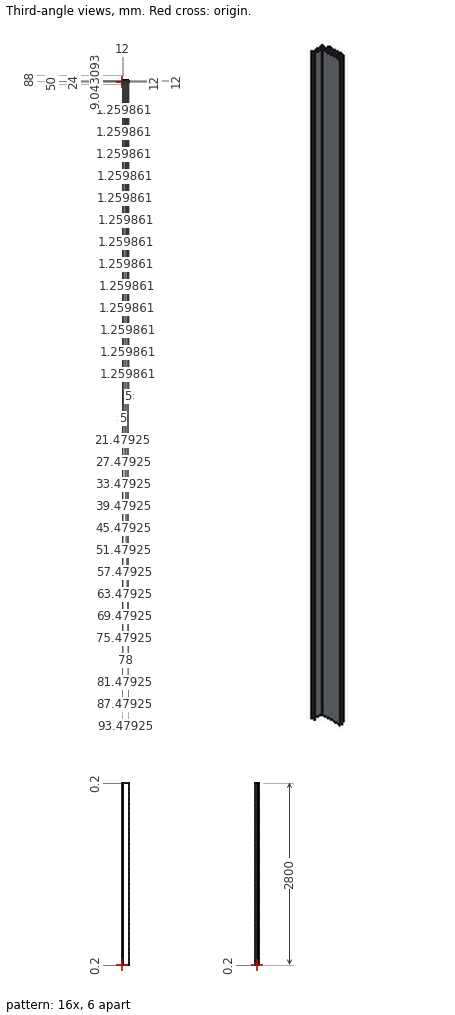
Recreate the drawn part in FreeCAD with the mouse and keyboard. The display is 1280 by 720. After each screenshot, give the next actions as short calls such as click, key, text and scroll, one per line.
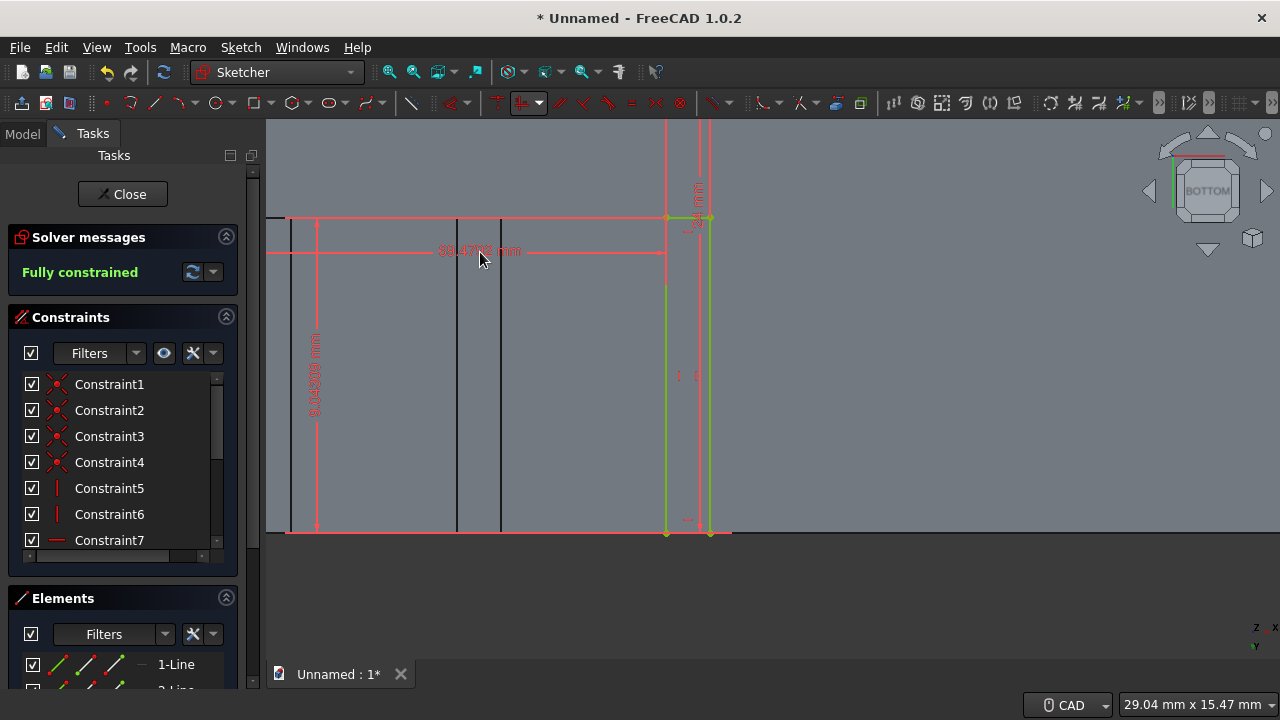
click(123, 194)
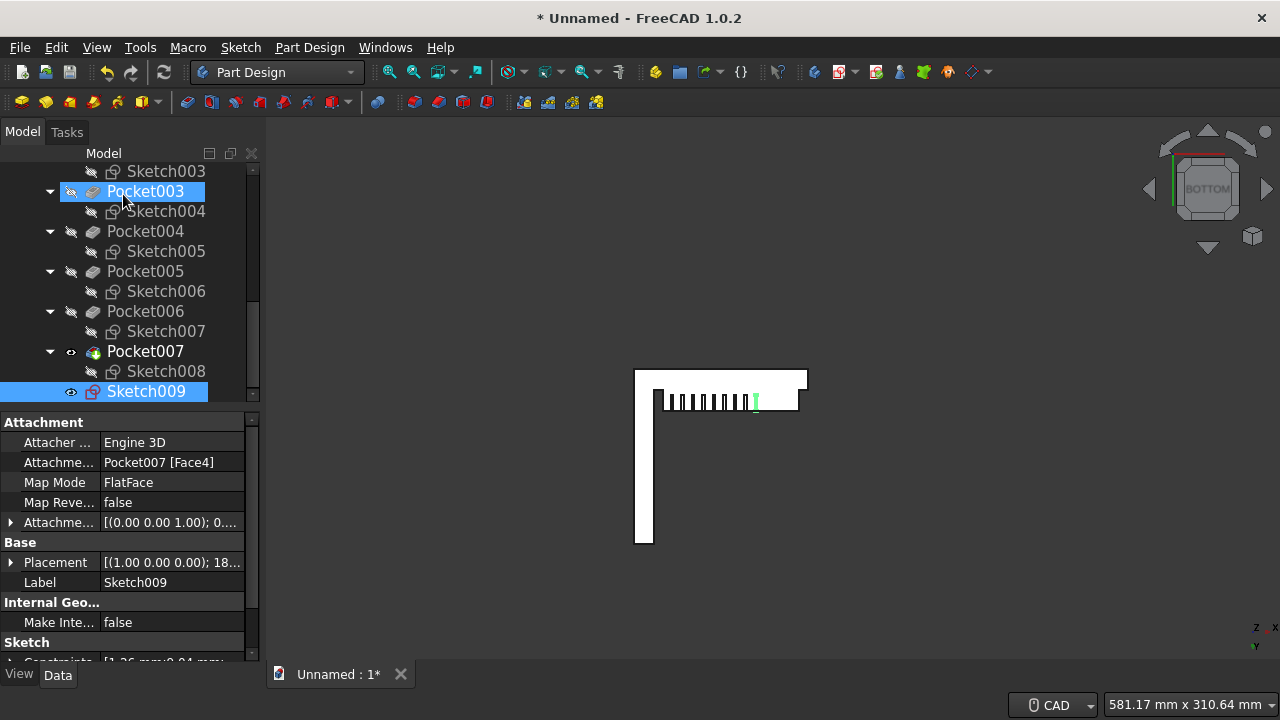
click(188, 102)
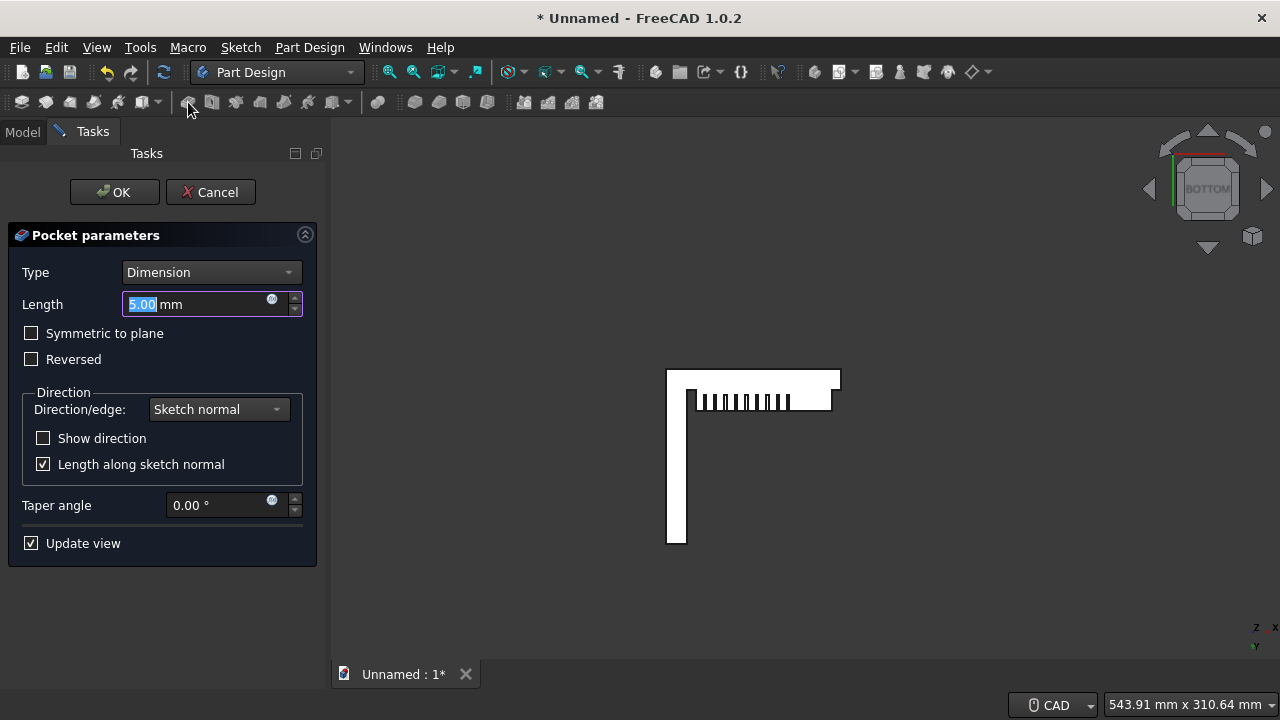
text(0.2)
key(Tab)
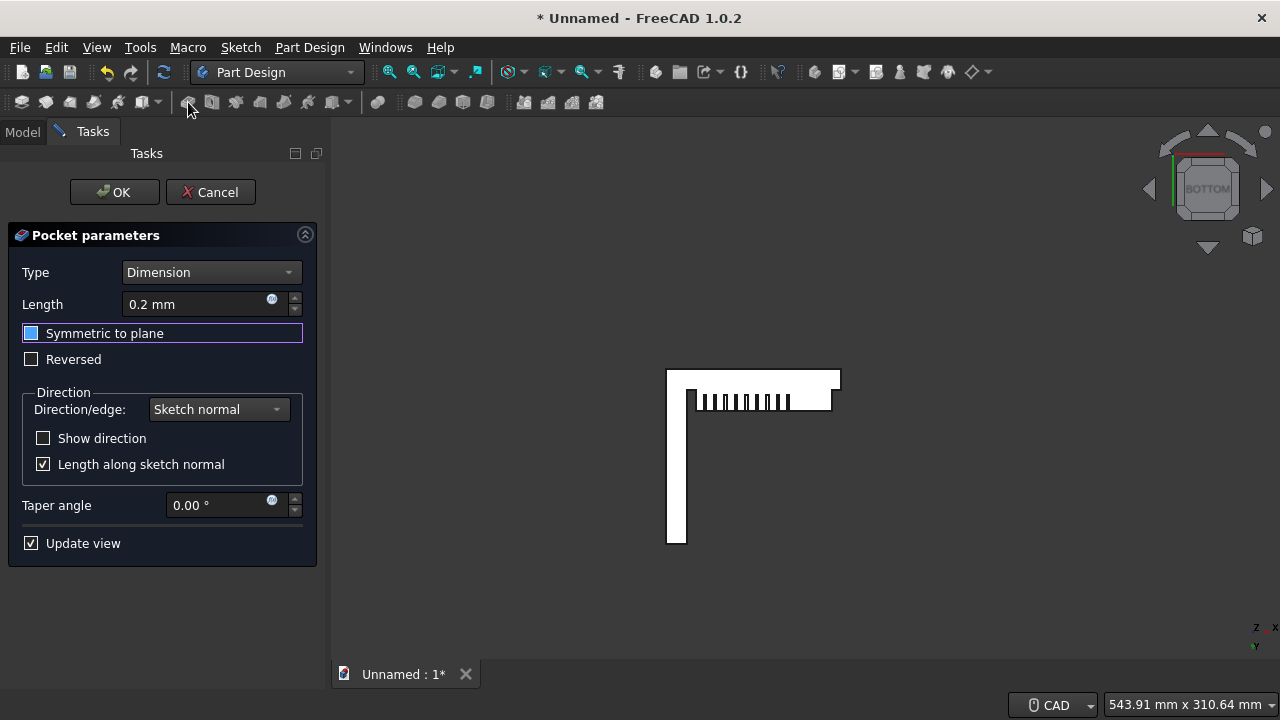
click(115, 192)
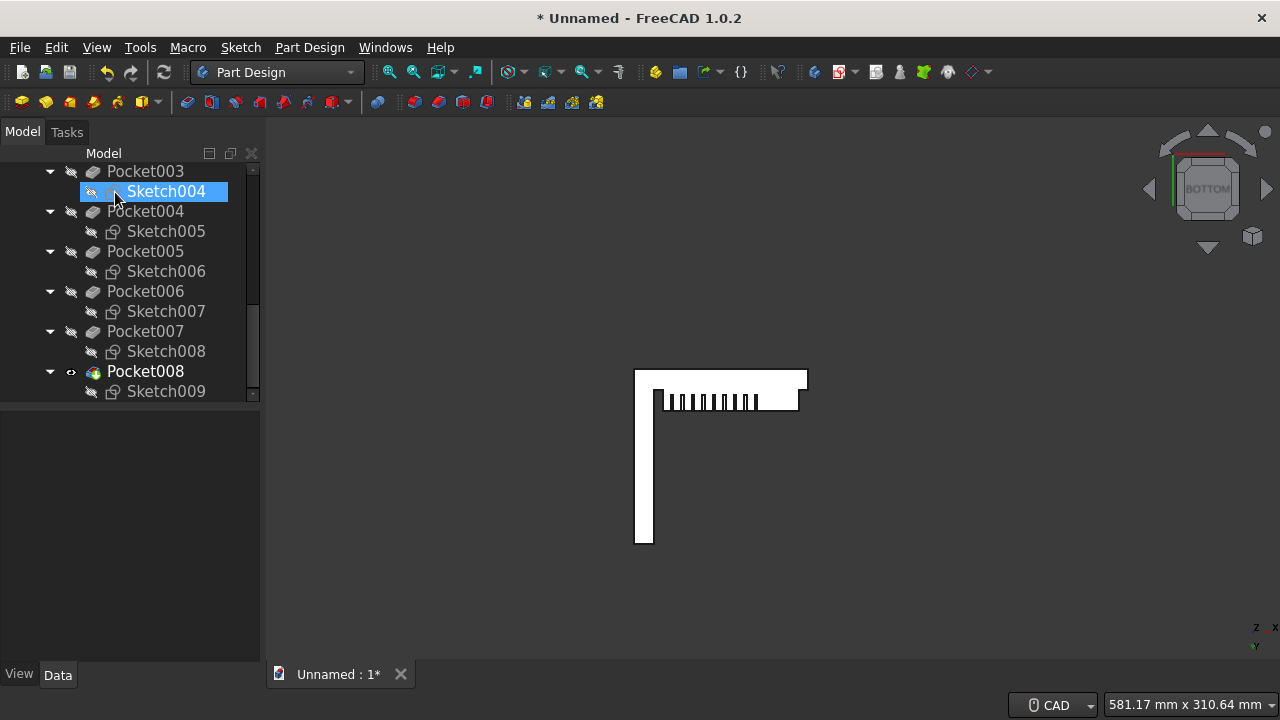
click(390, 72)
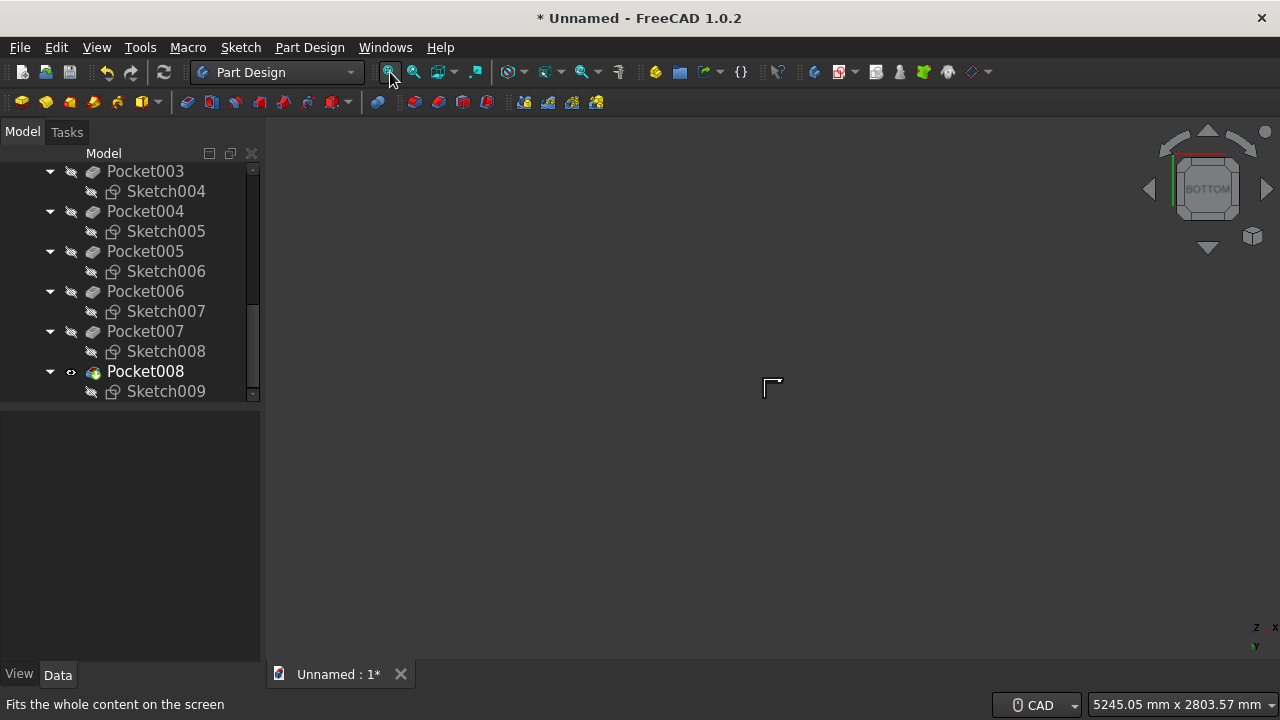
click(840, 72)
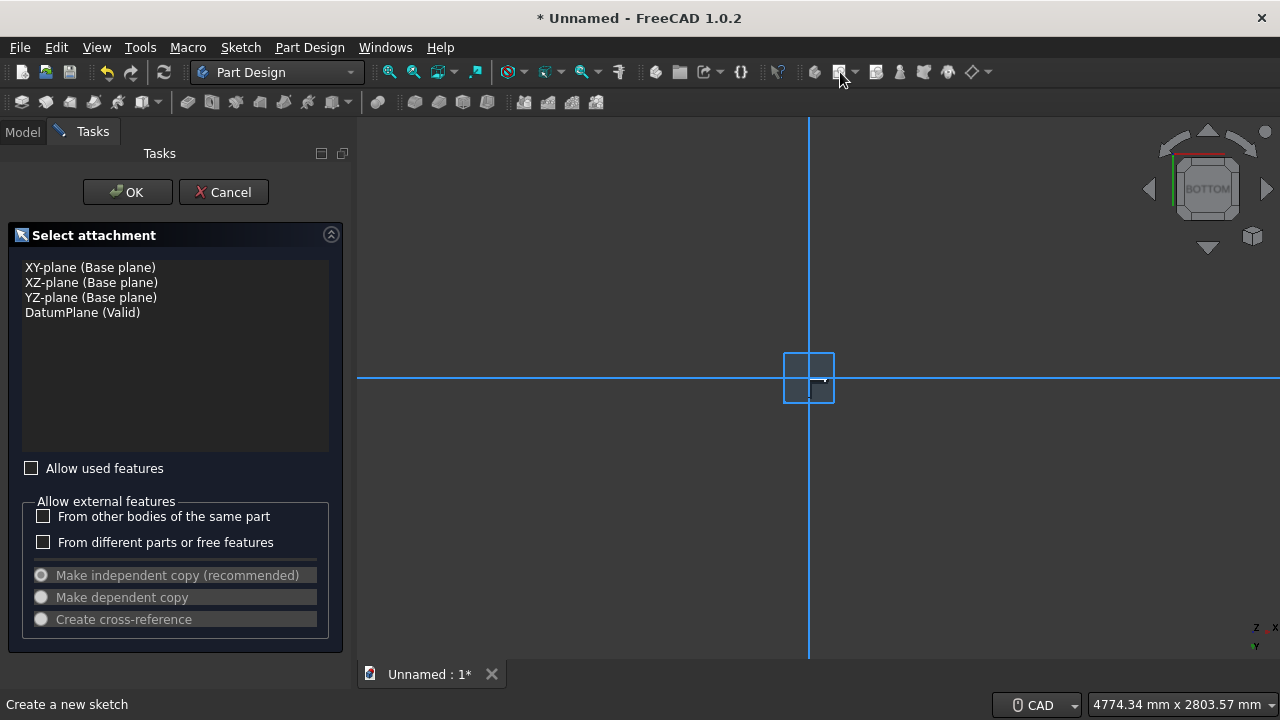
click(82, 268)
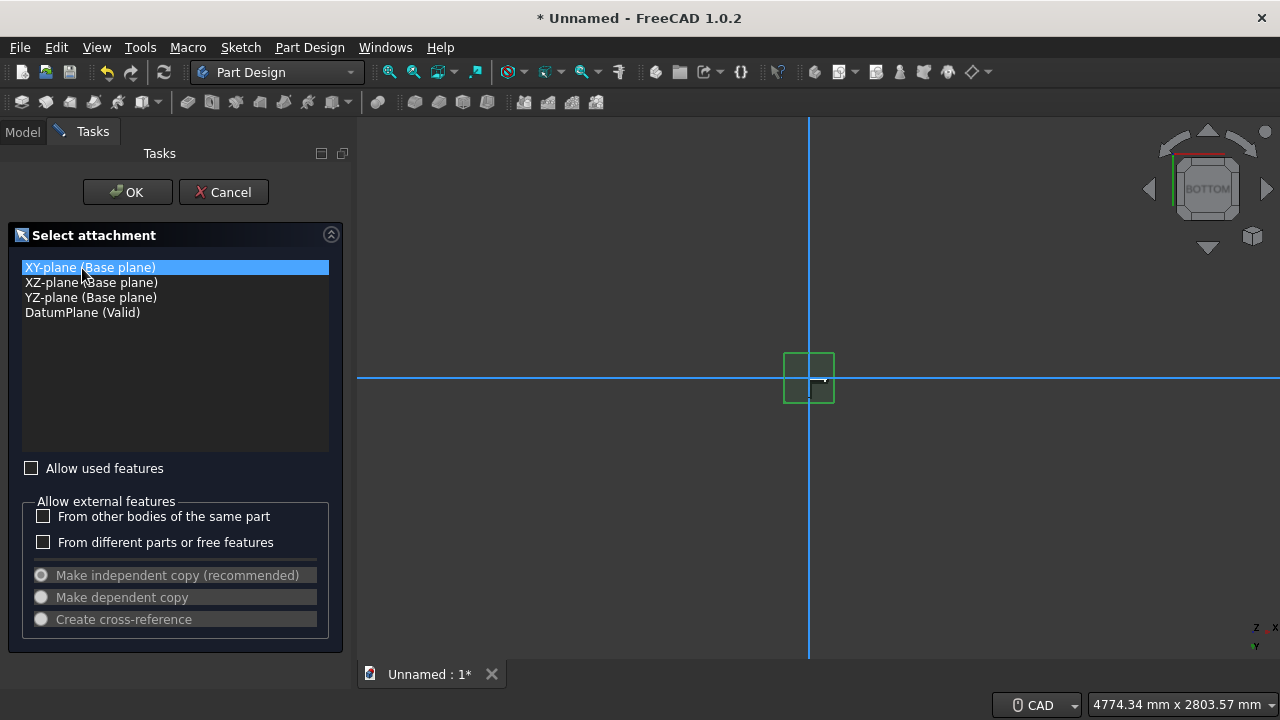
click(128, 192)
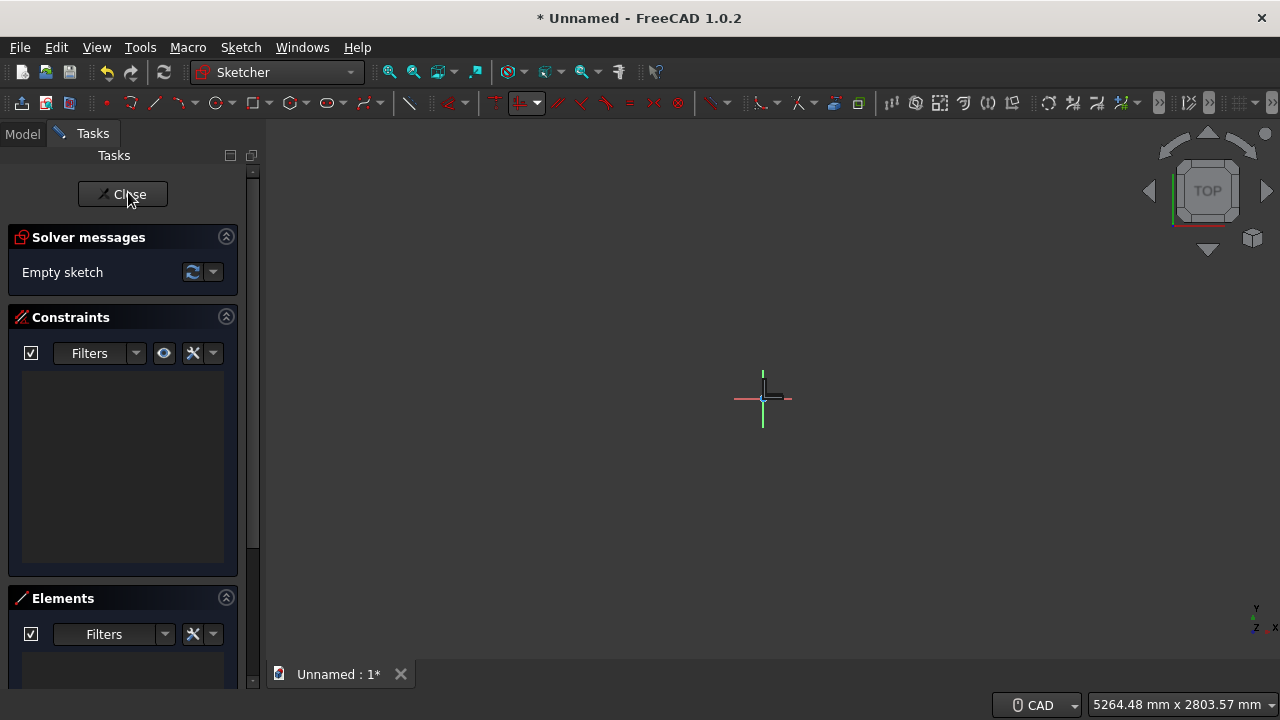
click(70, 104)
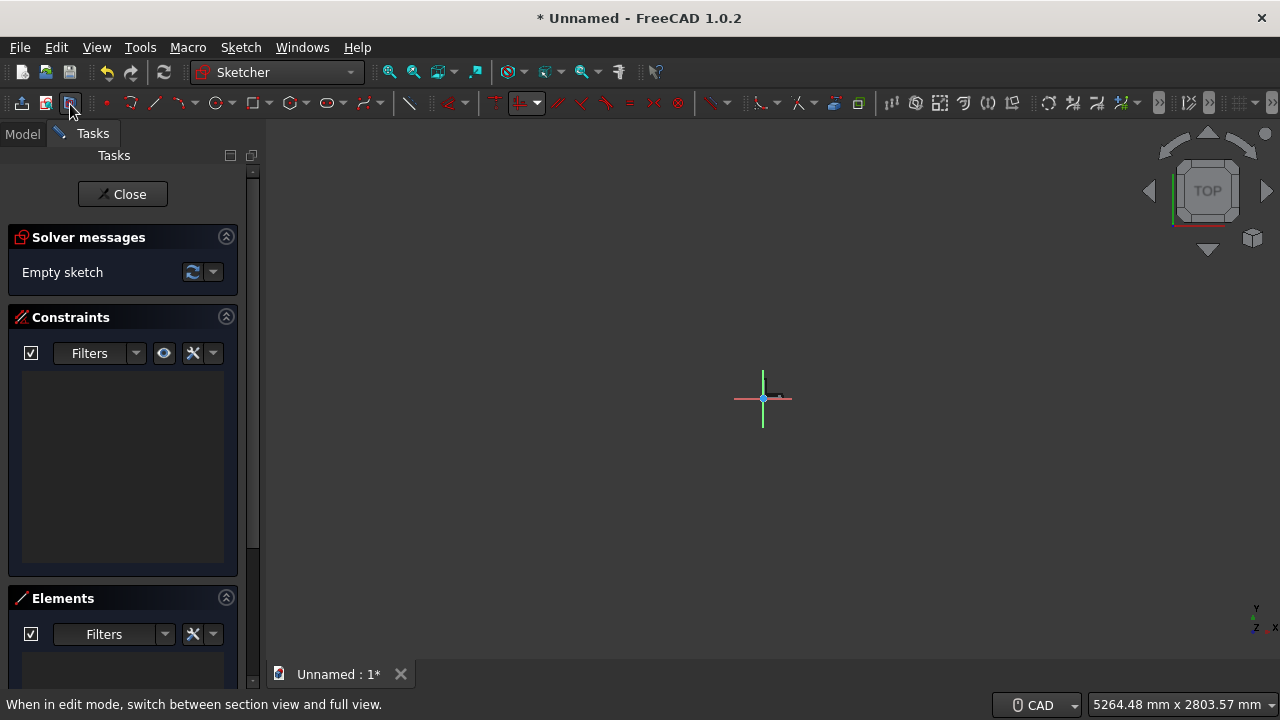
scroll(782, 395, up, 15)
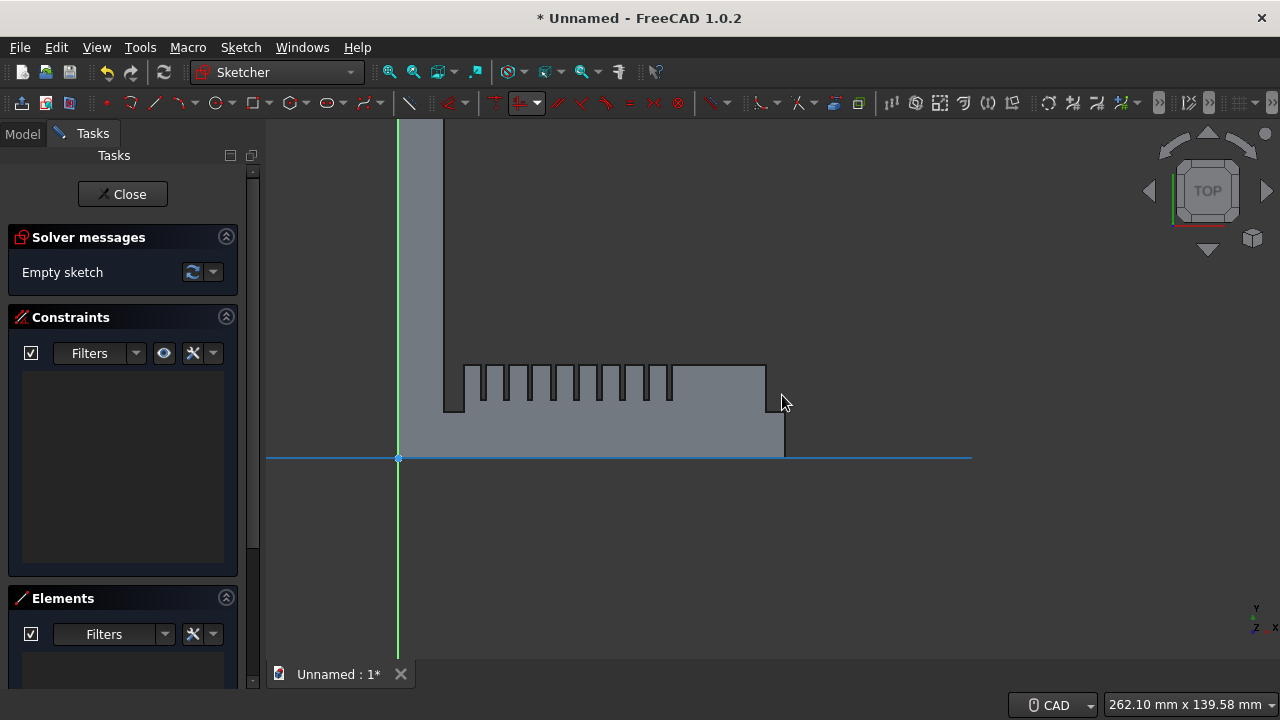
scroll(691, 382, up, 11)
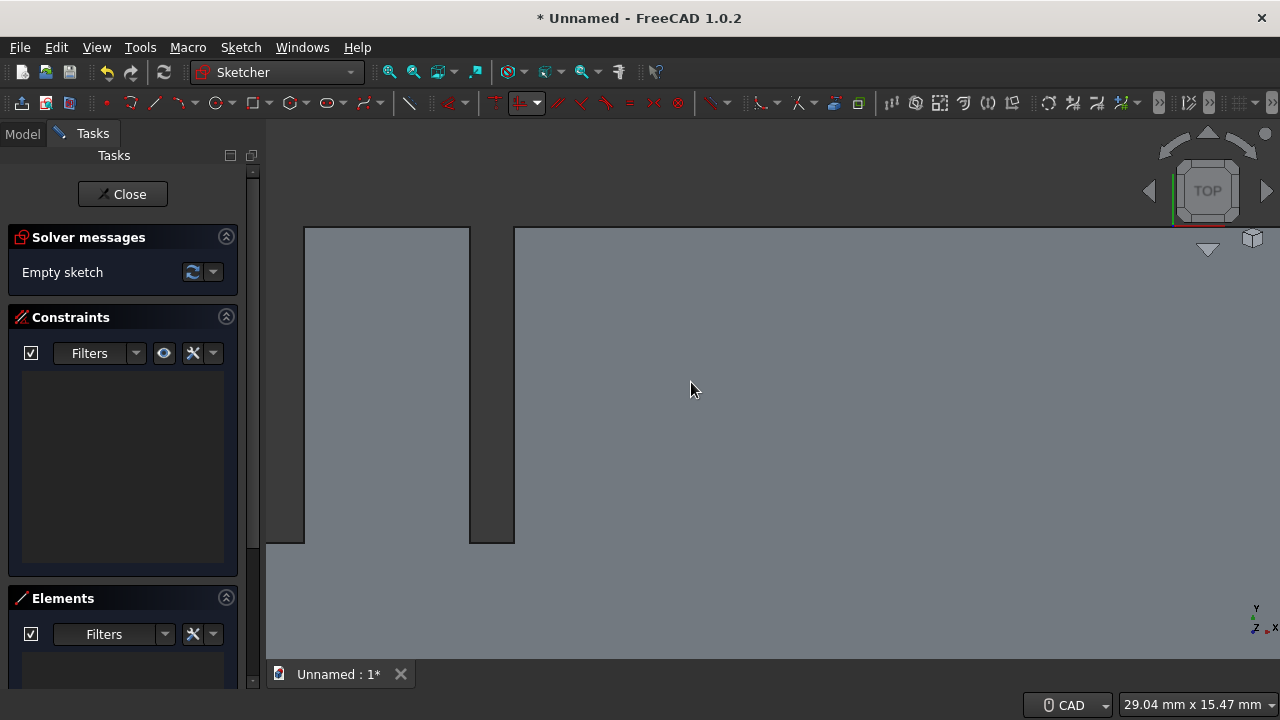
click(254, 104)